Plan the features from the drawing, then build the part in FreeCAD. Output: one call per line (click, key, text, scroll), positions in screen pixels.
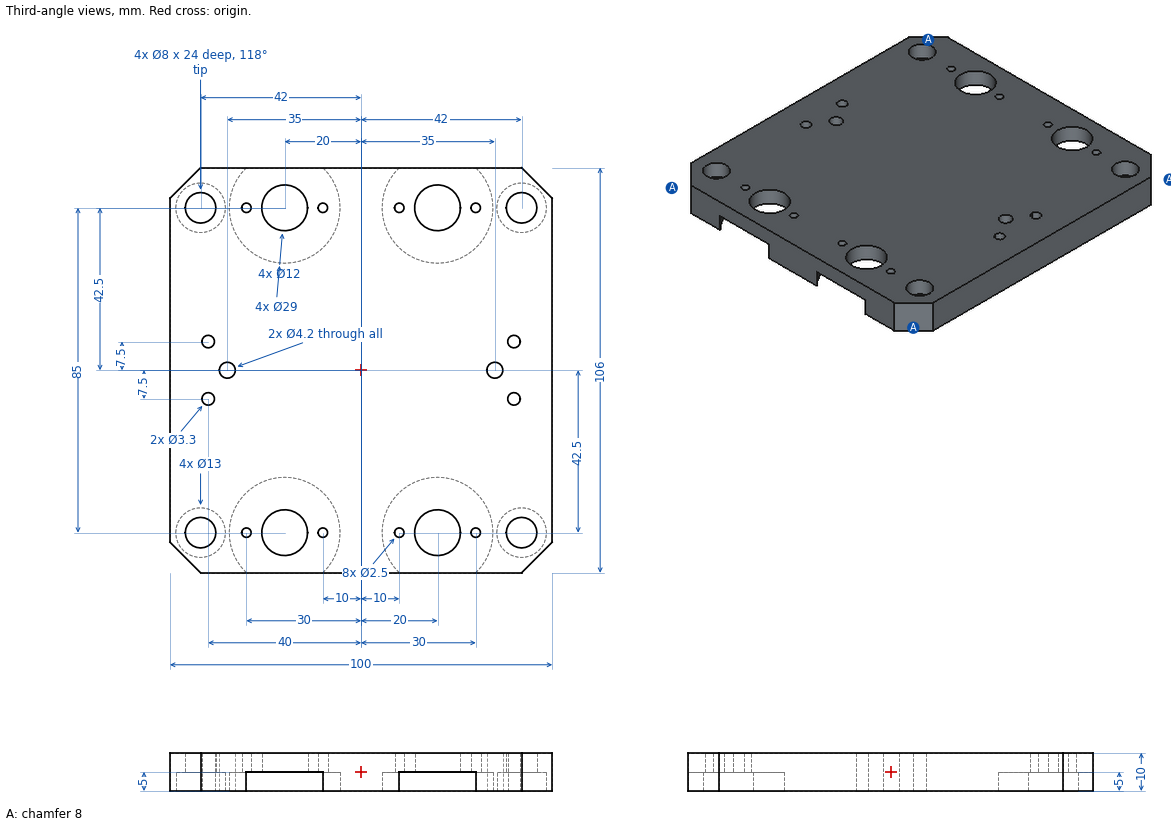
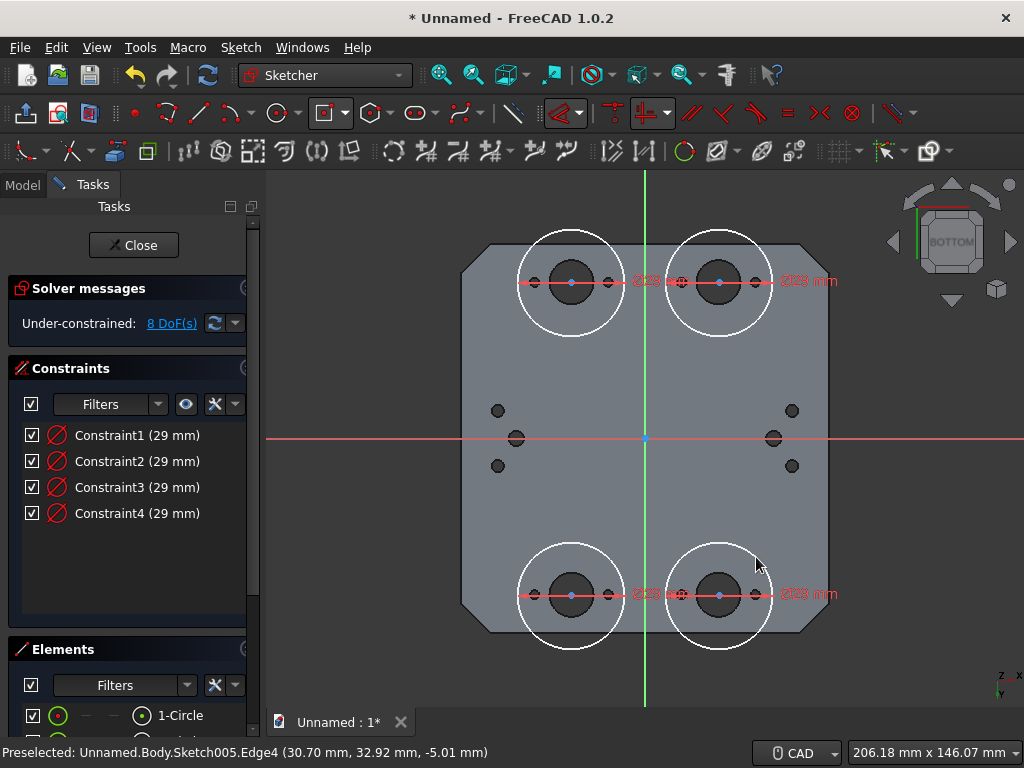
click(571, 596)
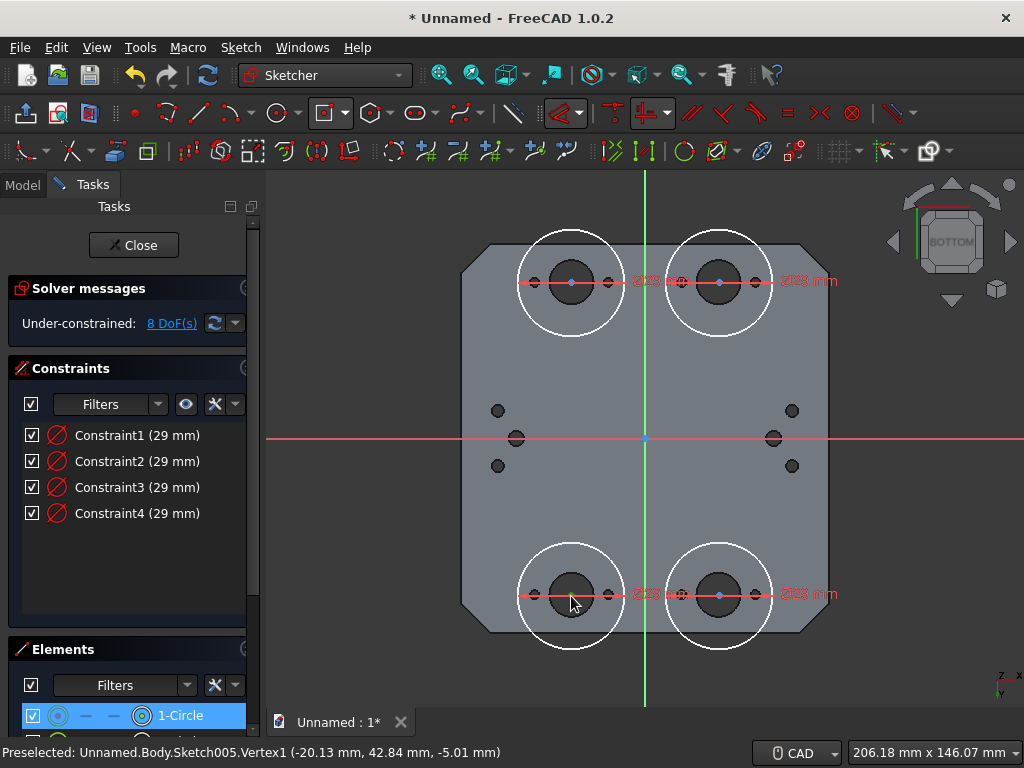
click(571, 283)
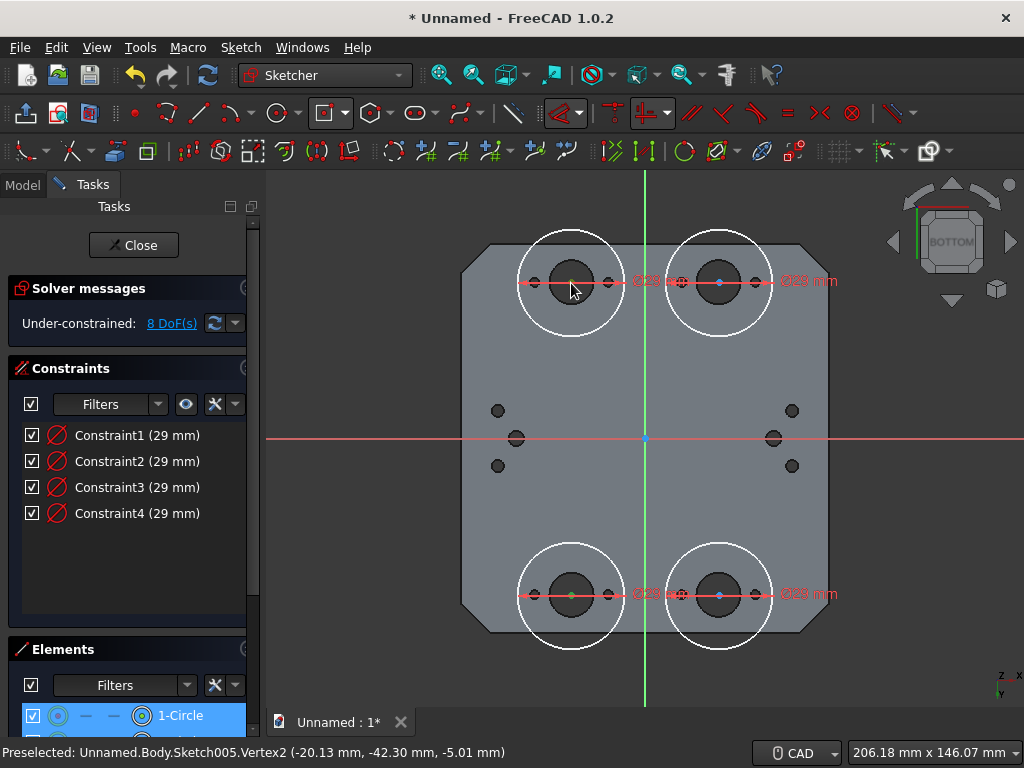
key(v)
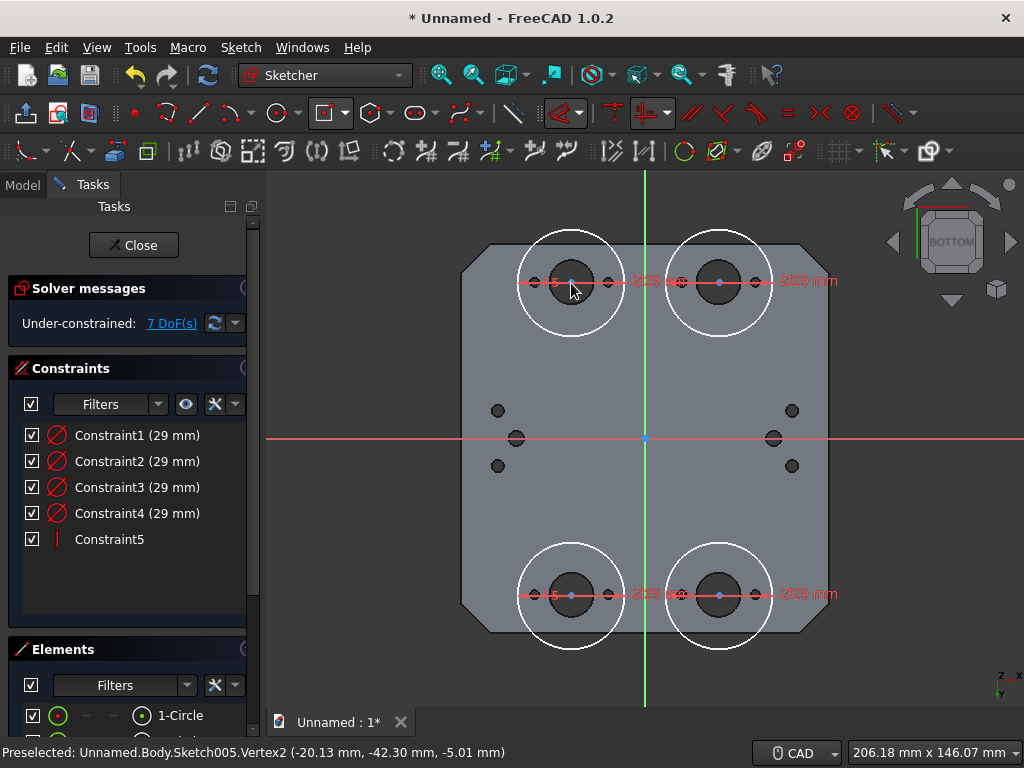
click(571, 283)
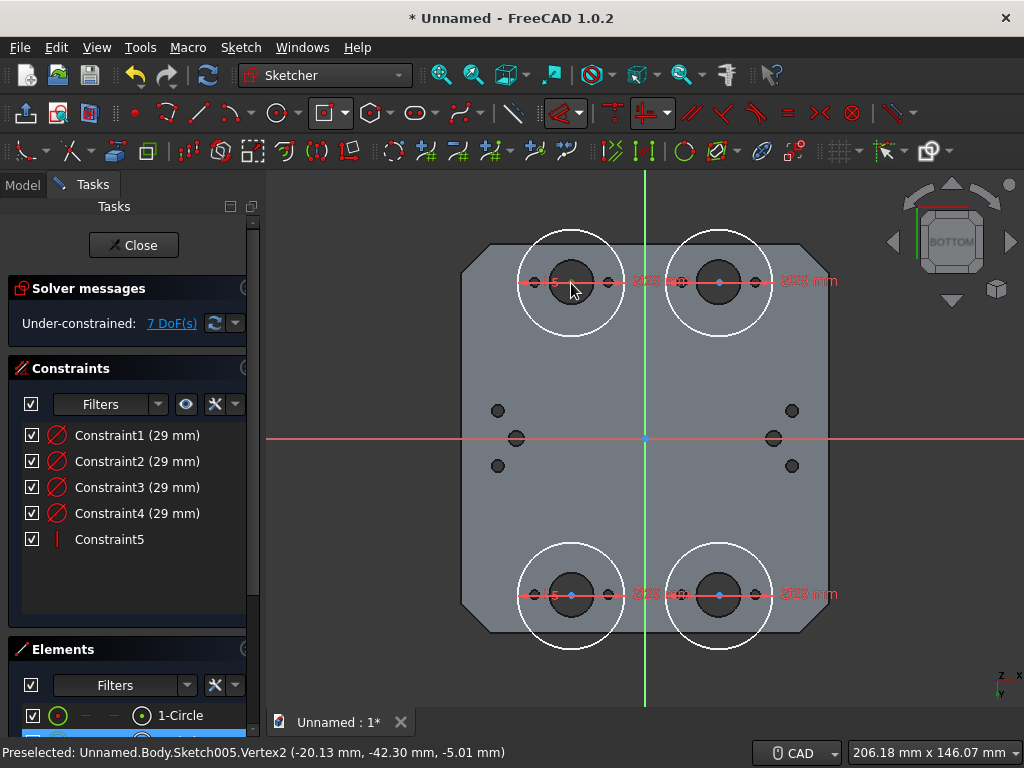
click(719, 283)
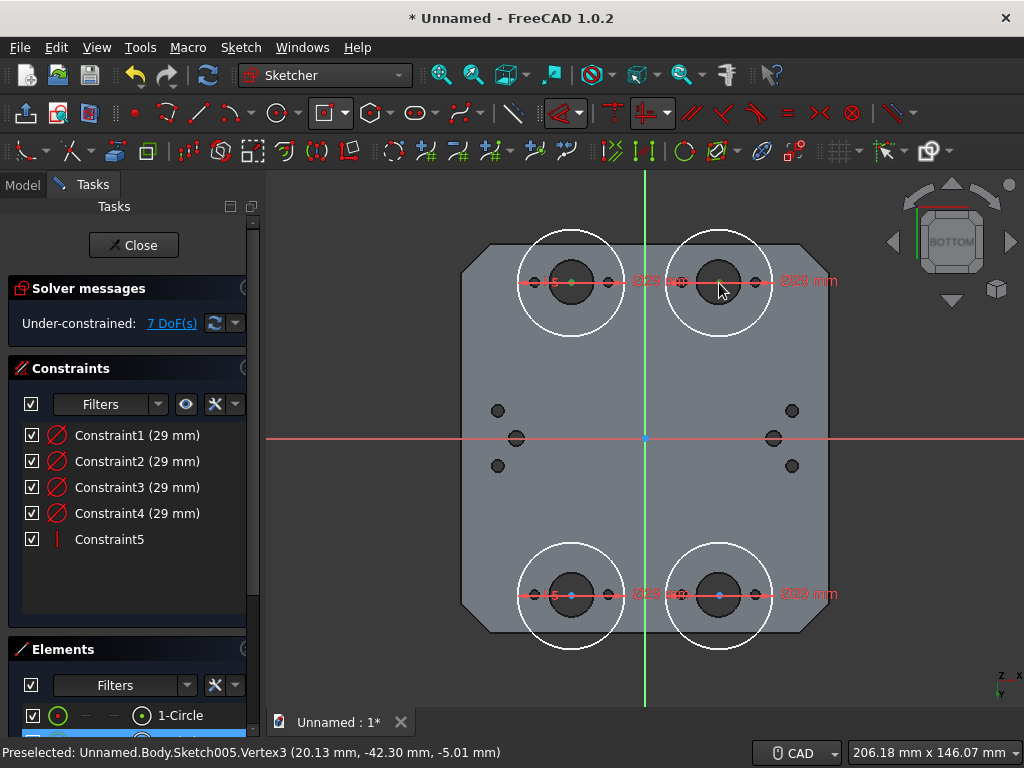
click(670, 114)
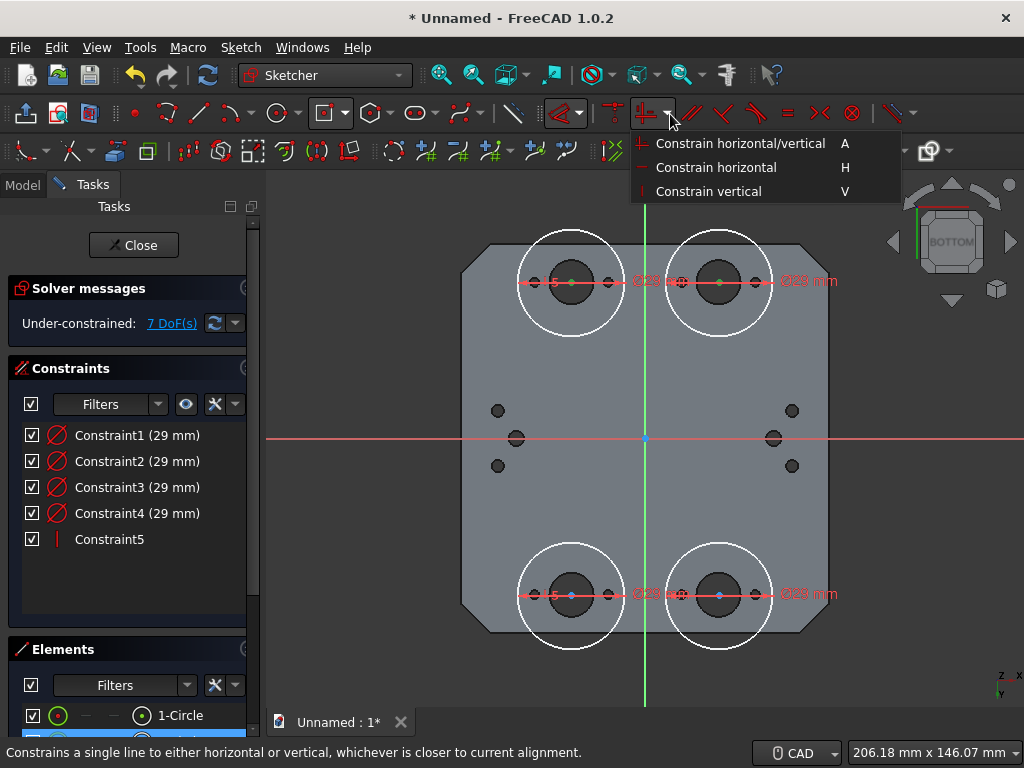
click(766, 167)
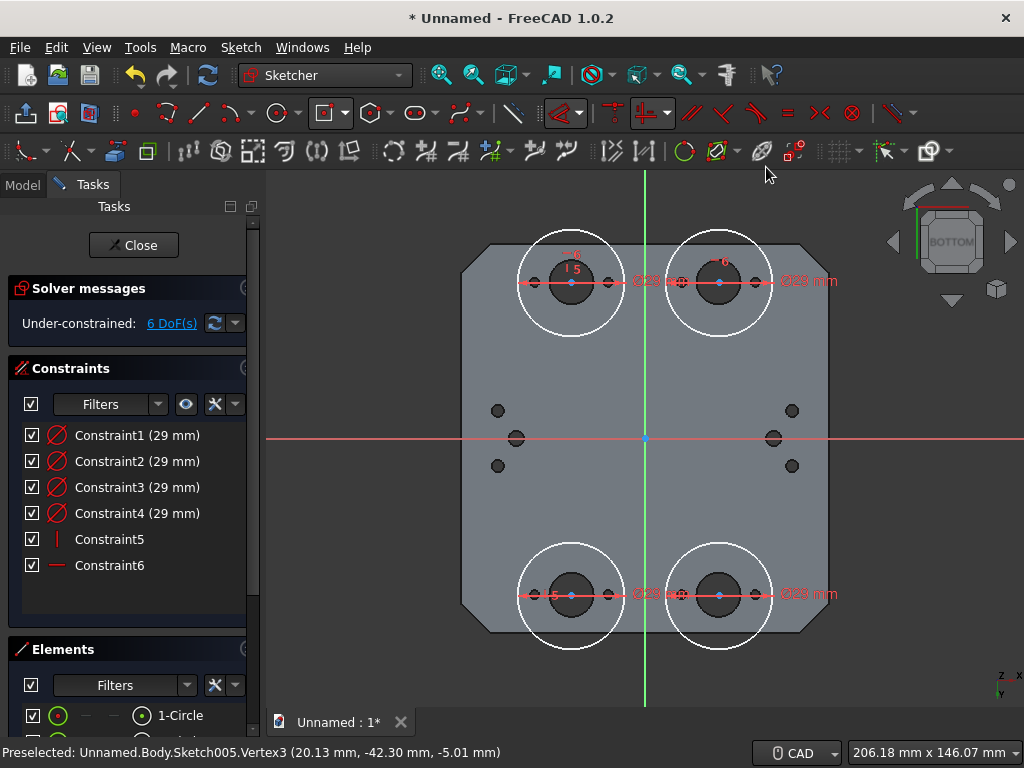
click(719, 283)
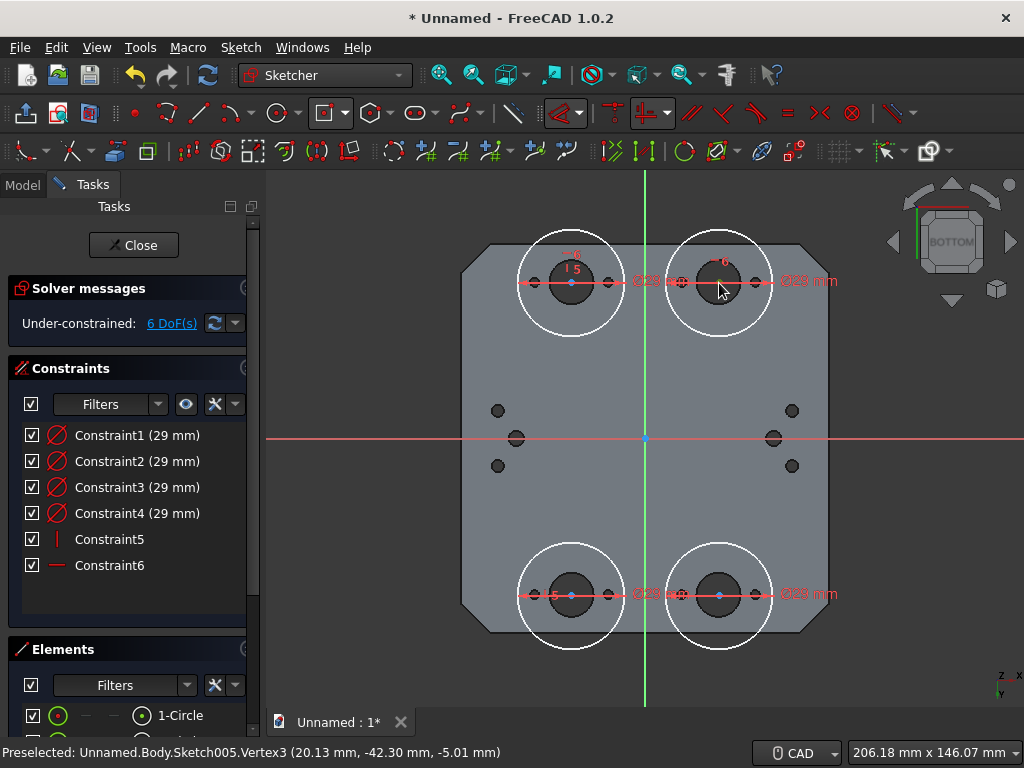
click(719, 596)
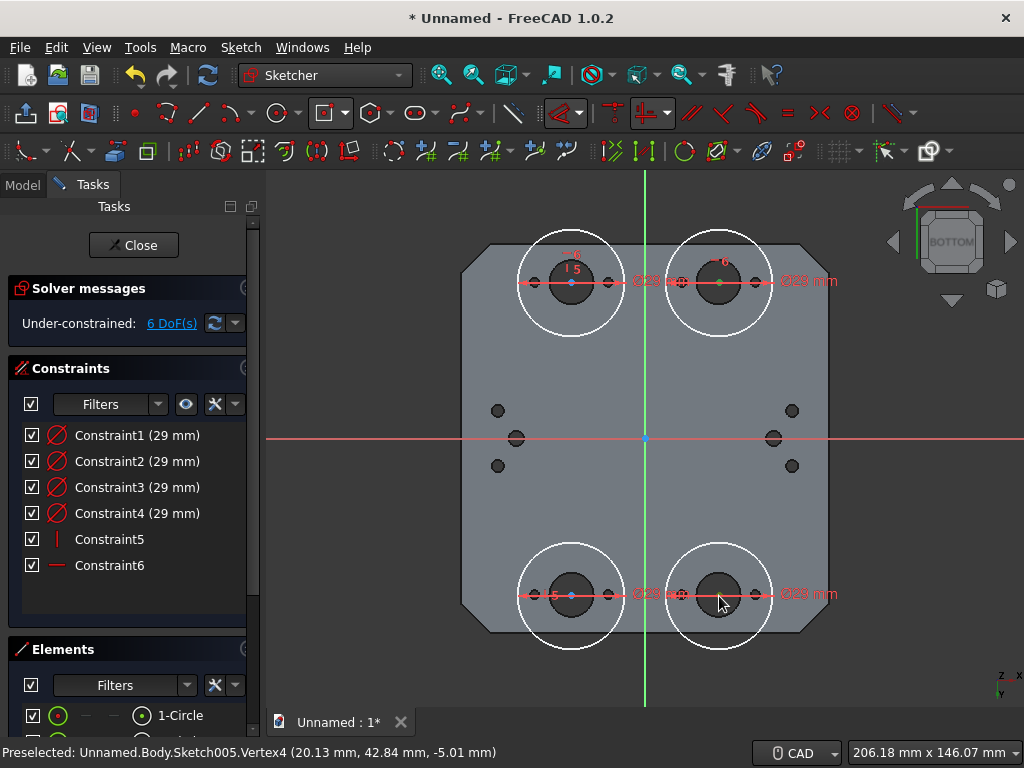
click(670, 114)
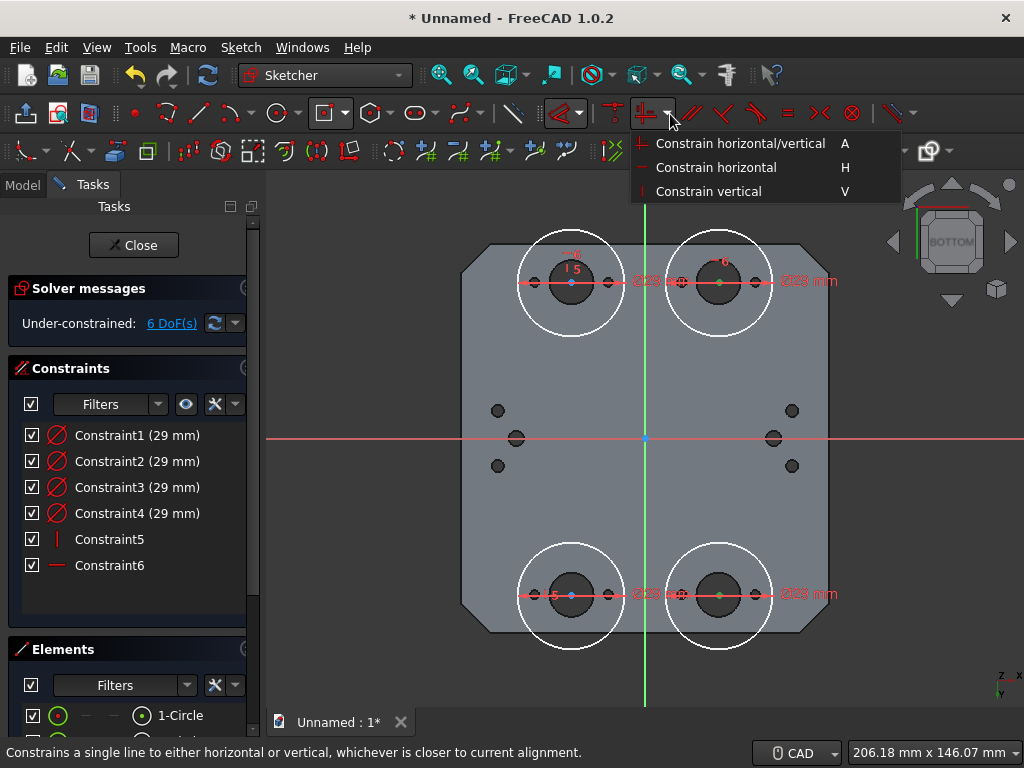
click(766, 191)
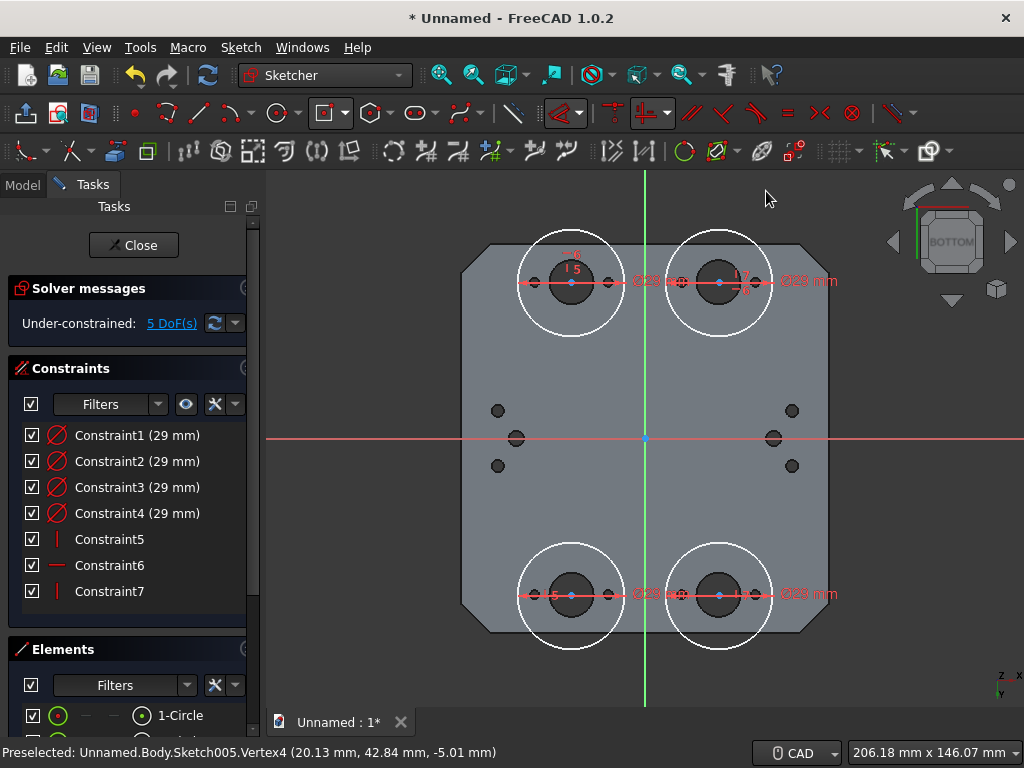
click(571, 596)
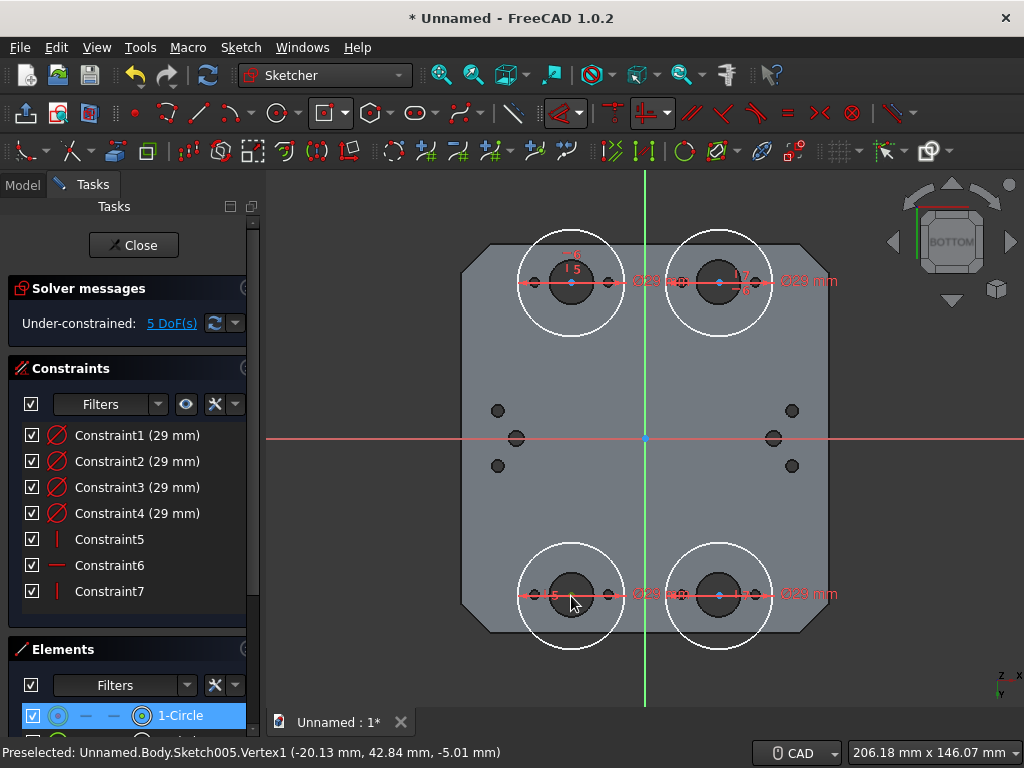
click(719, 596)